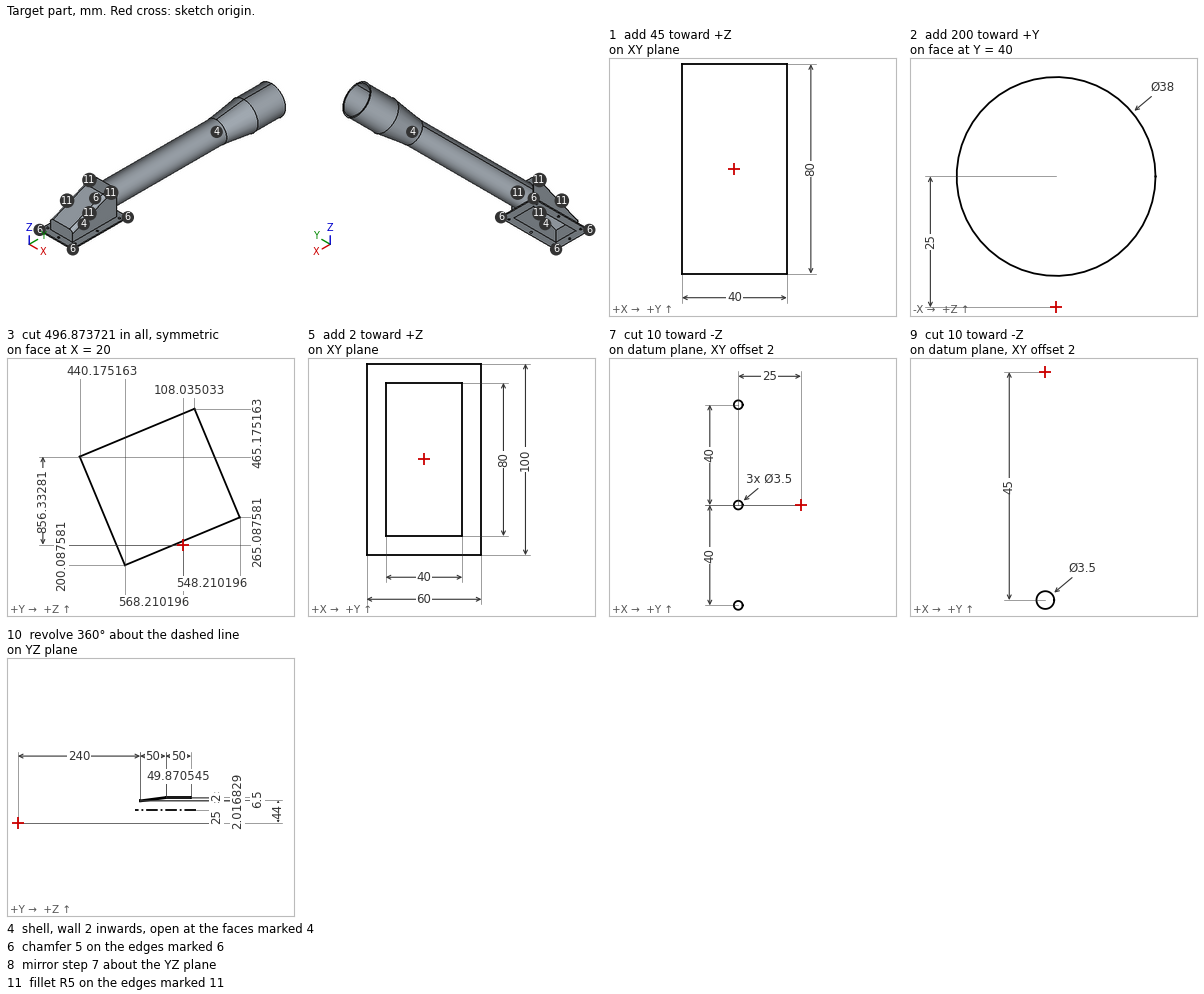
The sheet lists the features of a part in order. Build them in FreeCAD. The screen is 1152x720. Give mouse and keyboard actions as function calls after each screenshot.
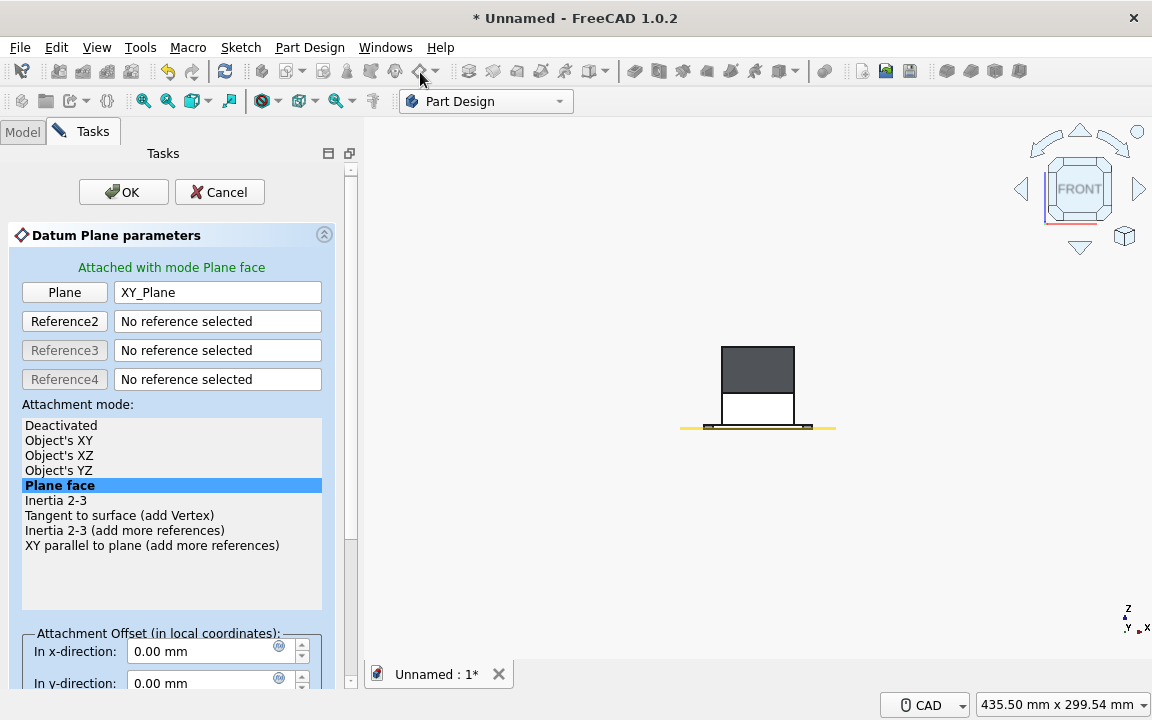
scroll(351, 426, down, 2)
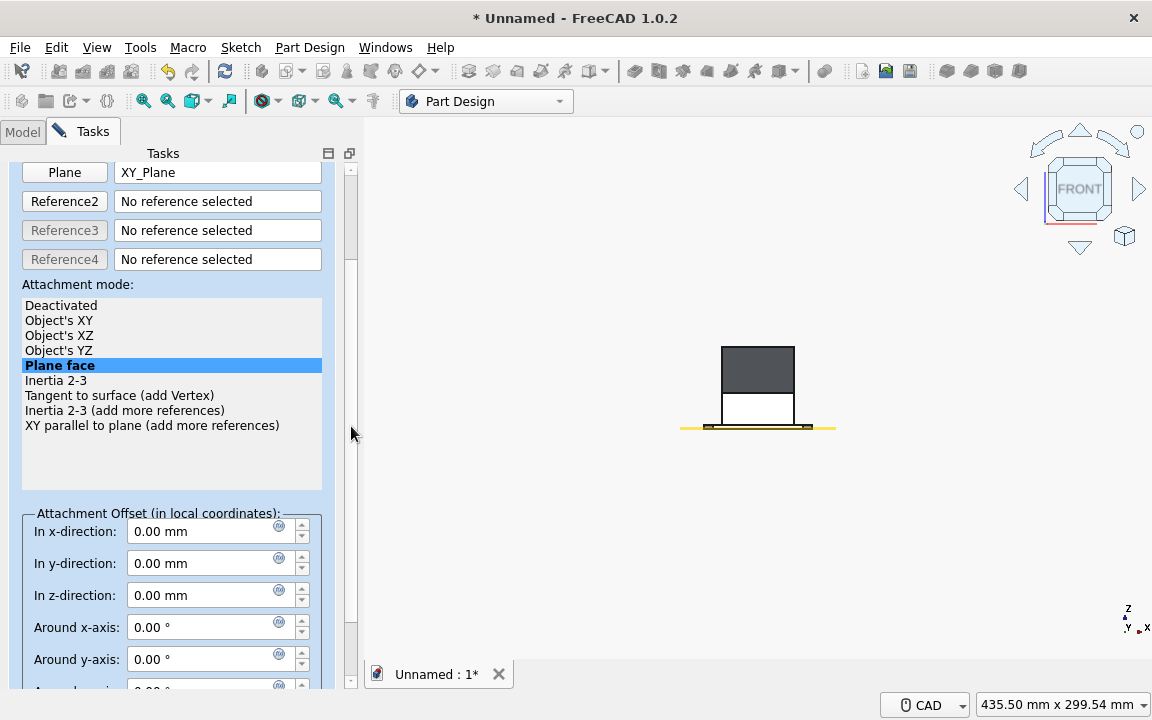
triple_click(210, 595)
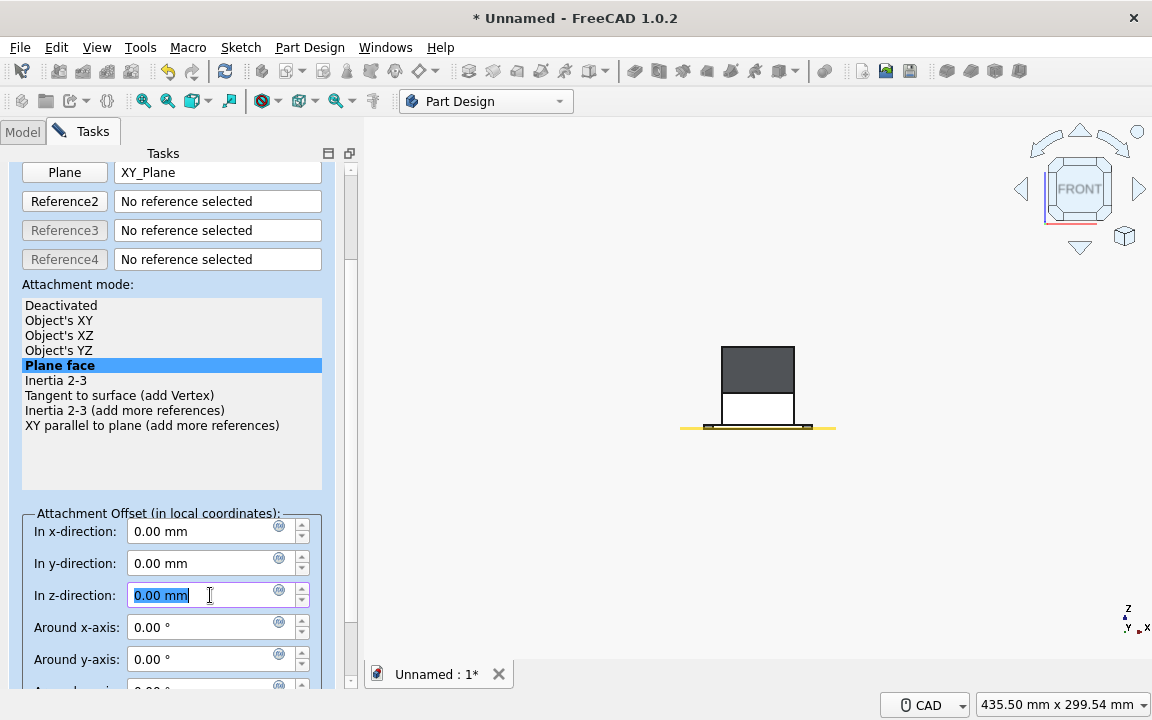
text(2)
key(Tab)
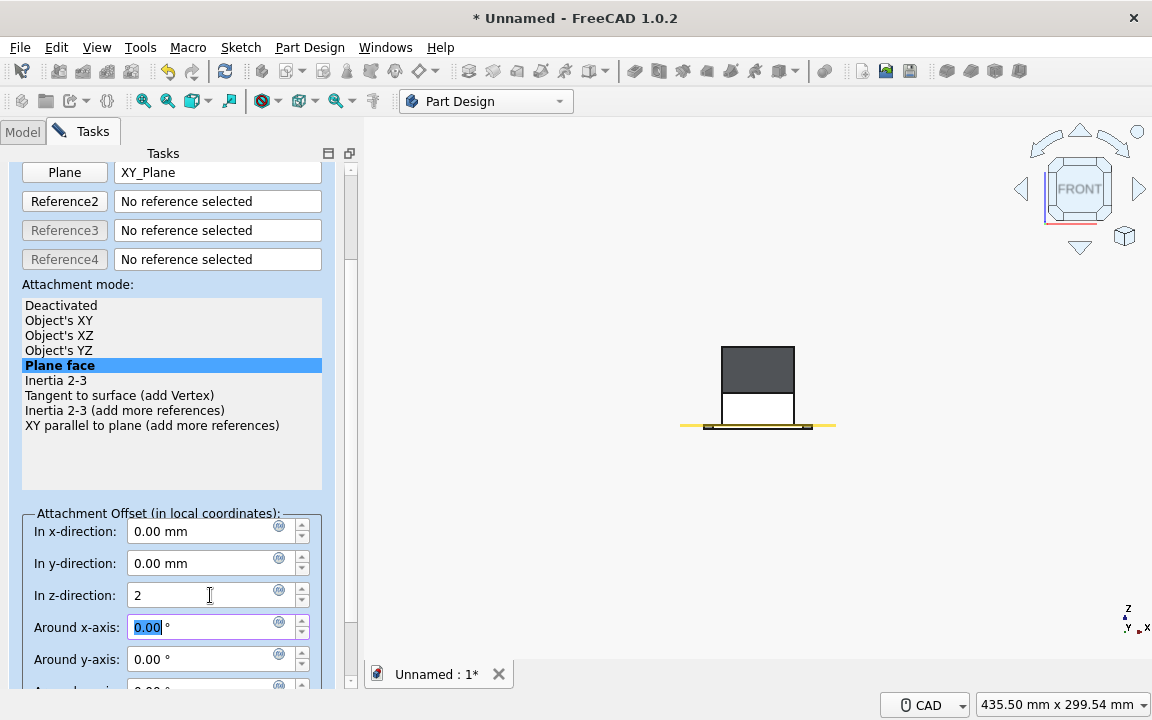
scroll(351, 426, up, 3)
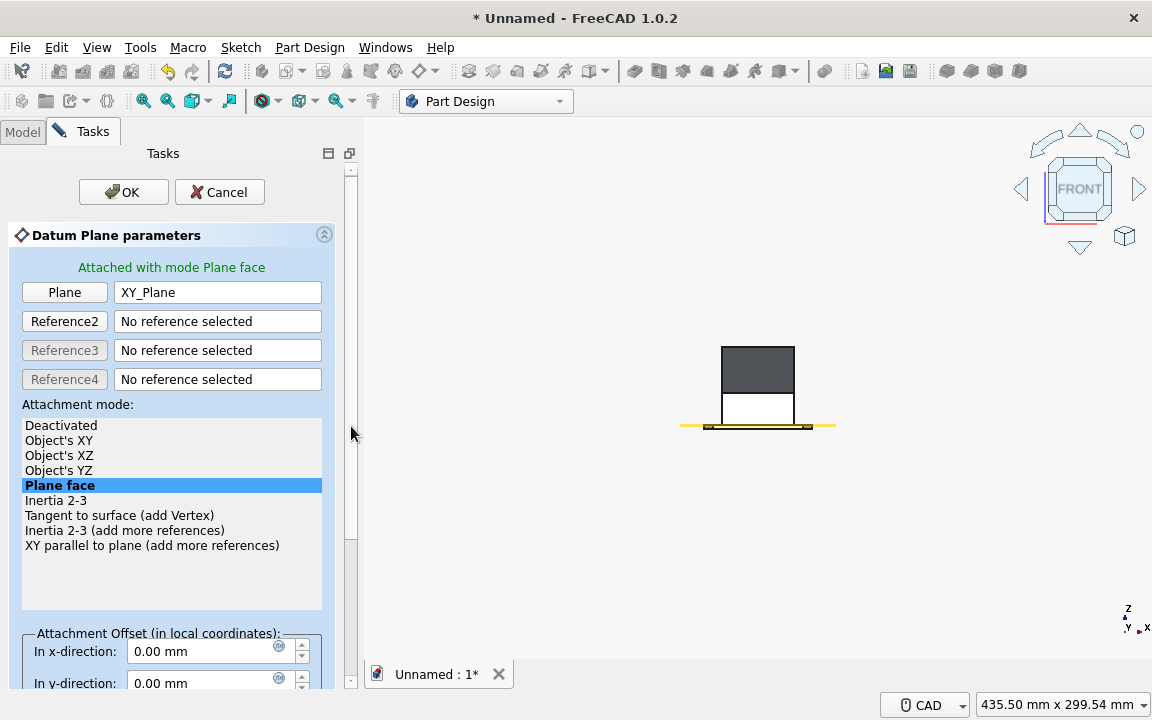
click(124, 192)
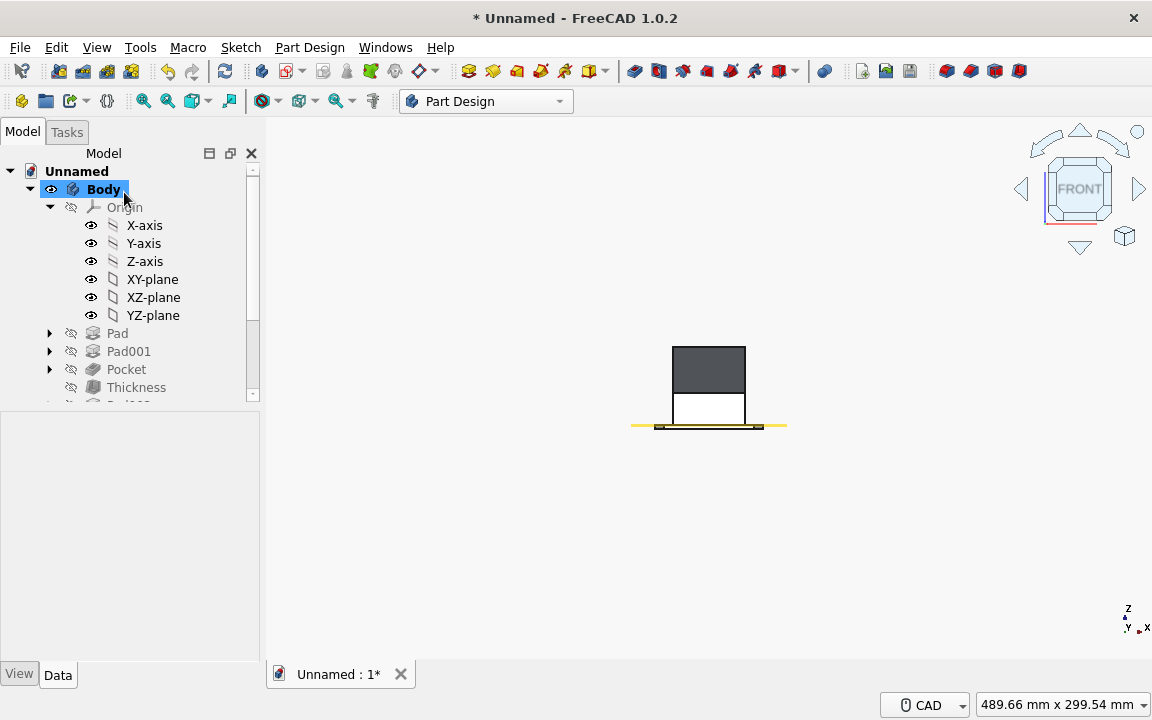
scroll(100, 275, down, 3)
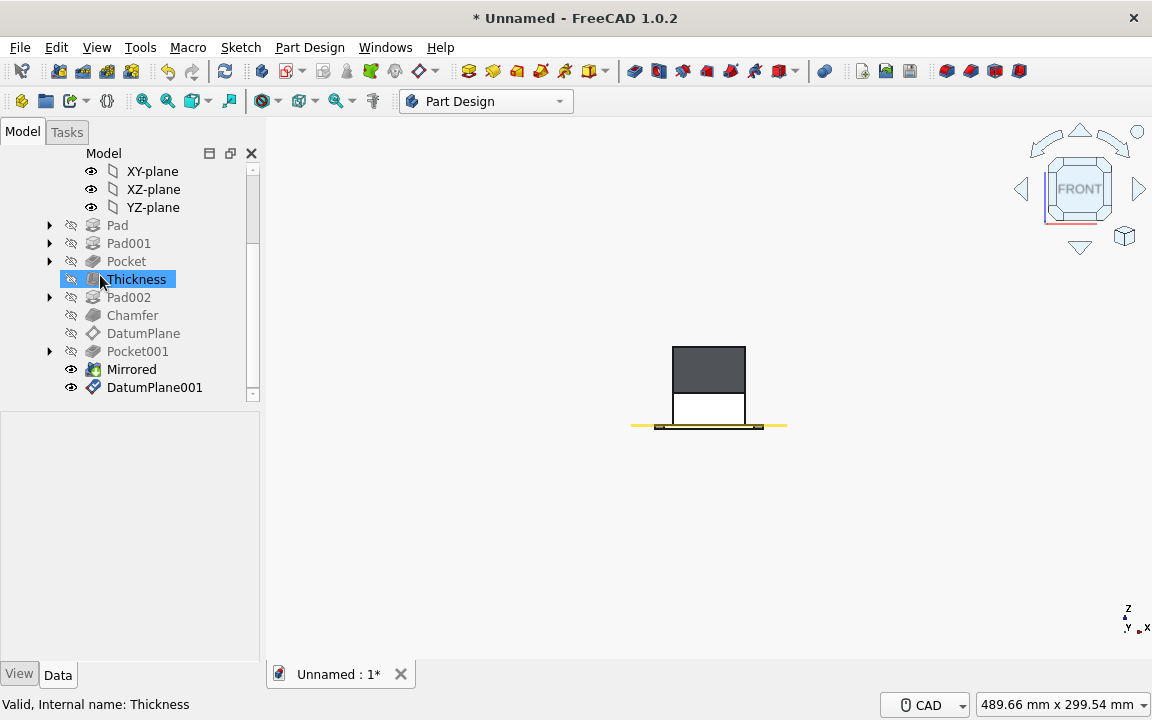
click(116, 387)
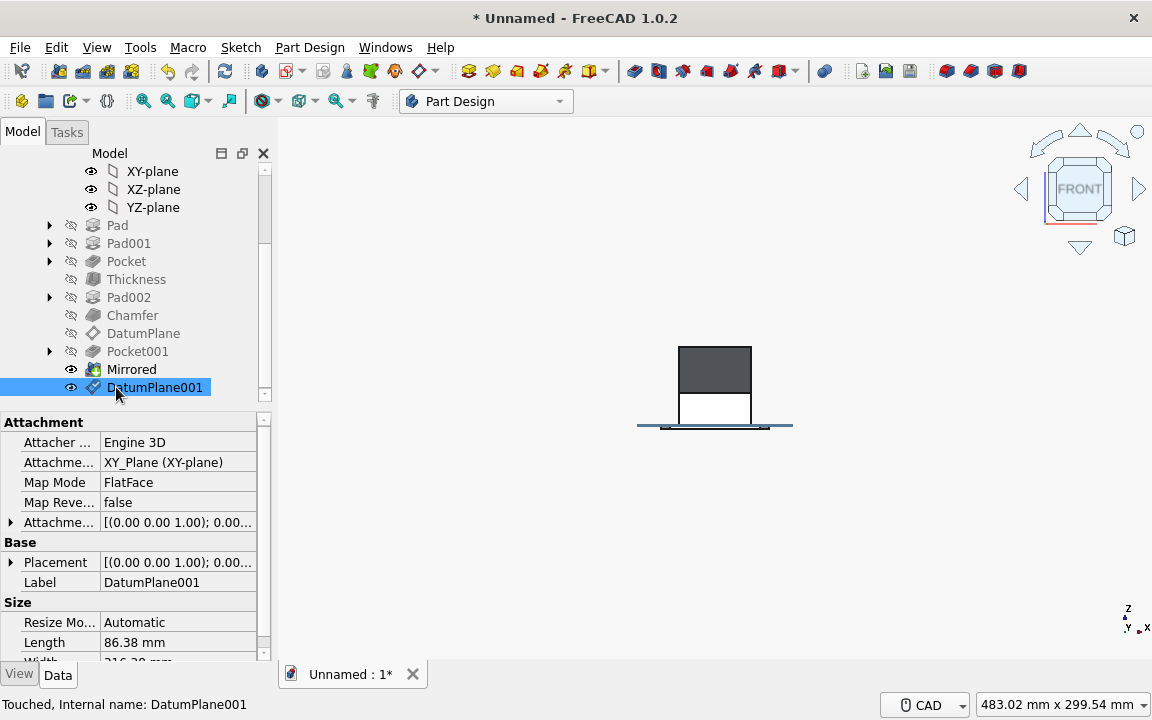
click(286, 72)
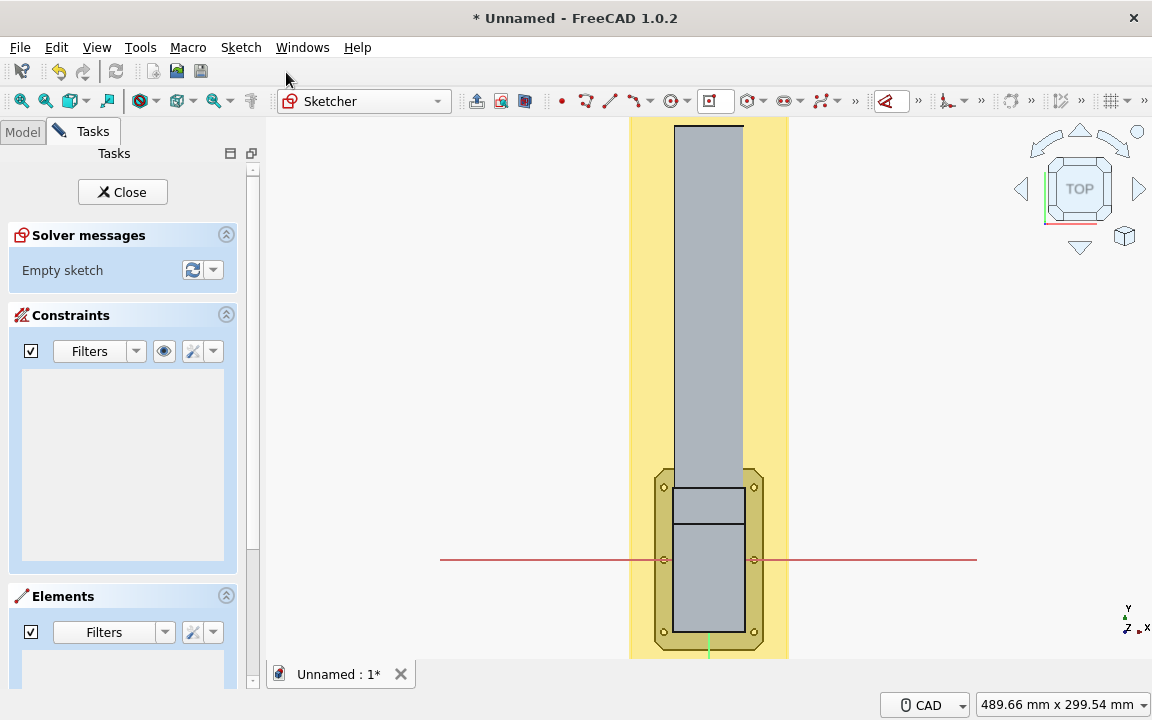
key(q)
key(s)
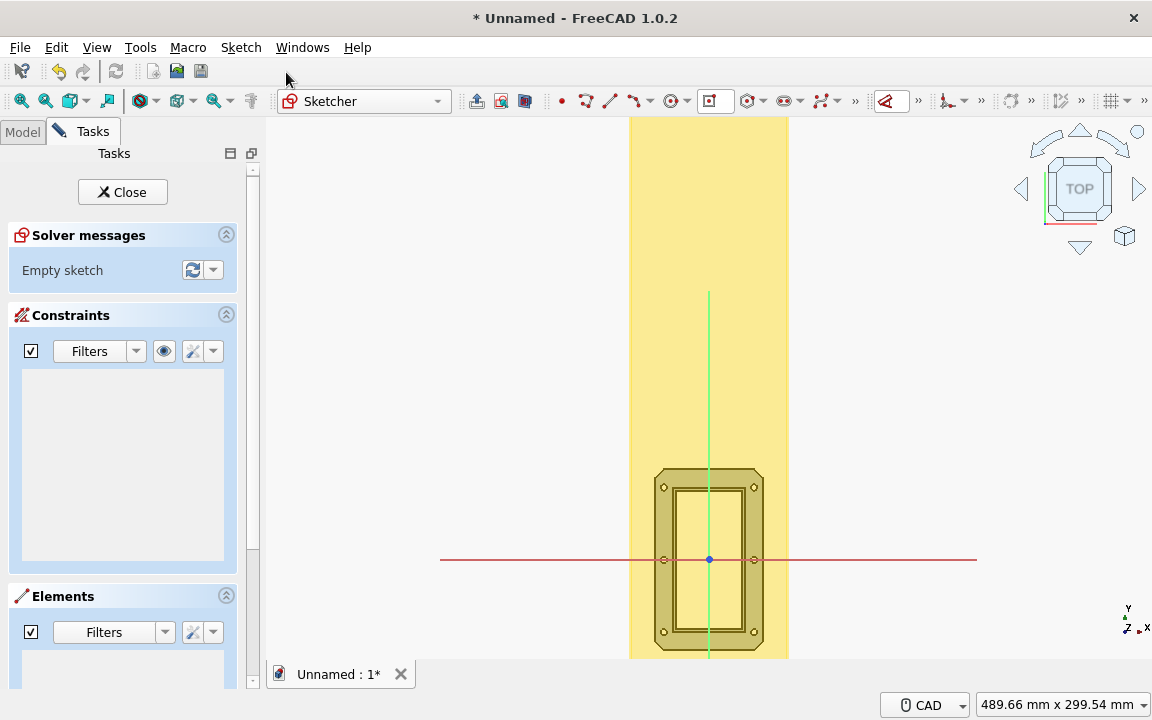
scroll(640, 388, down, 5)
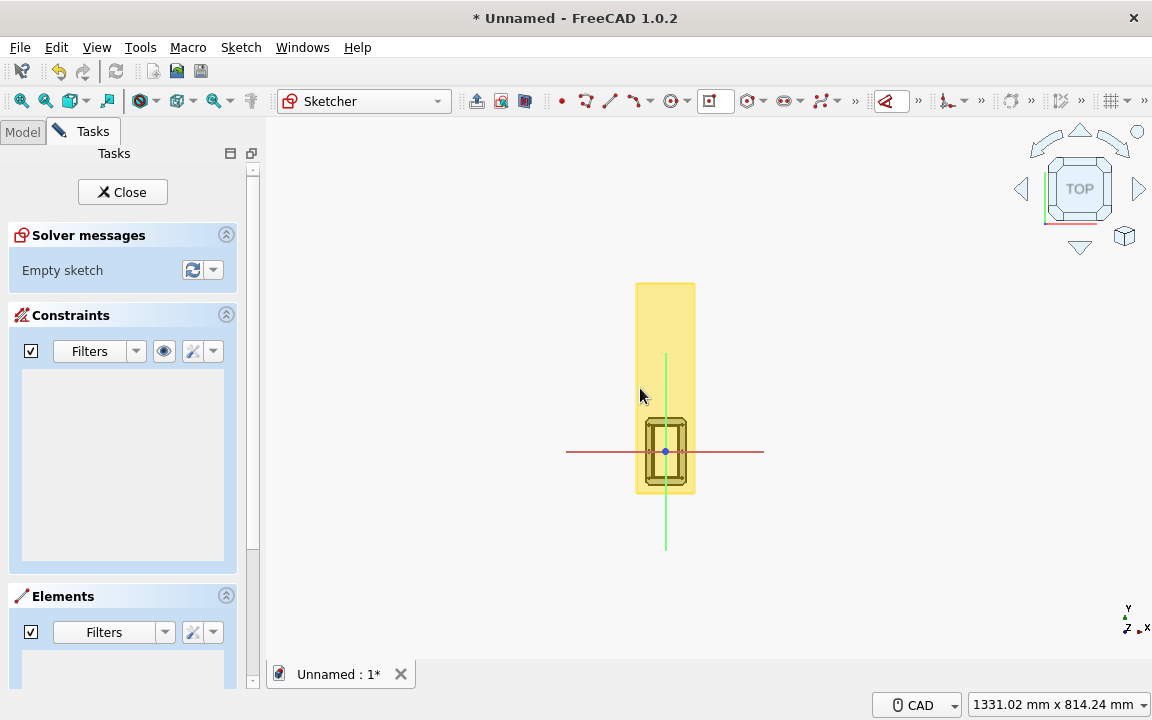
scroll(667, 486, up, 15)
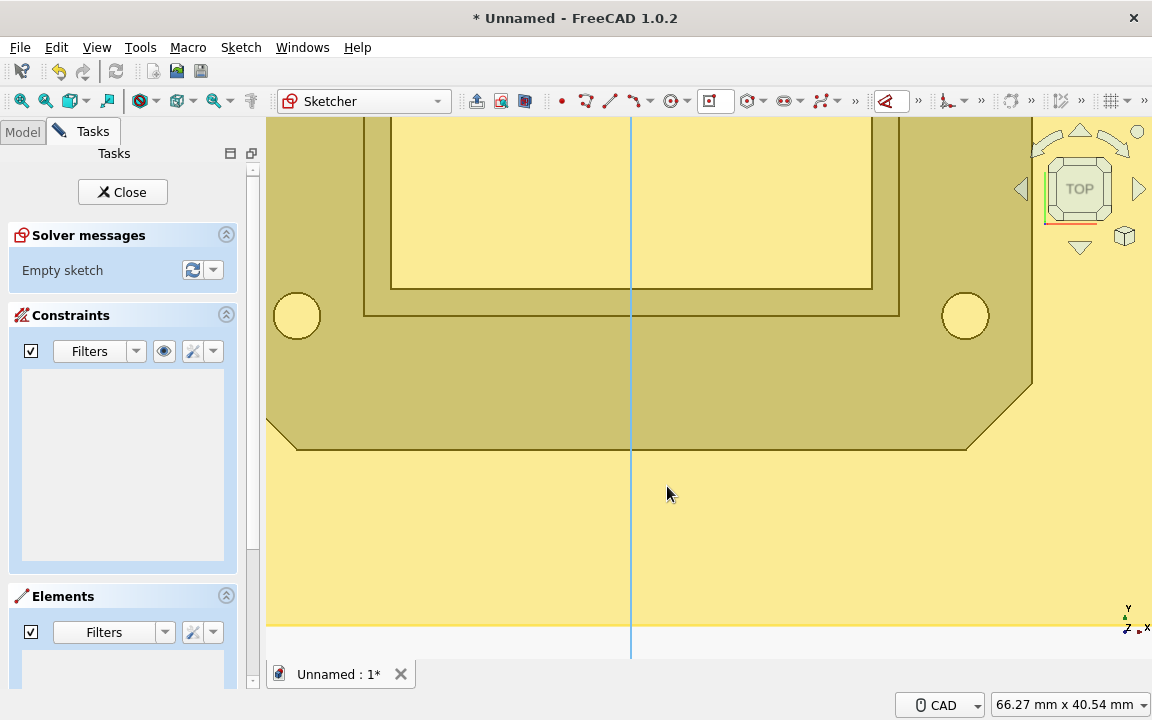
scroll(630, 382, up, 10)